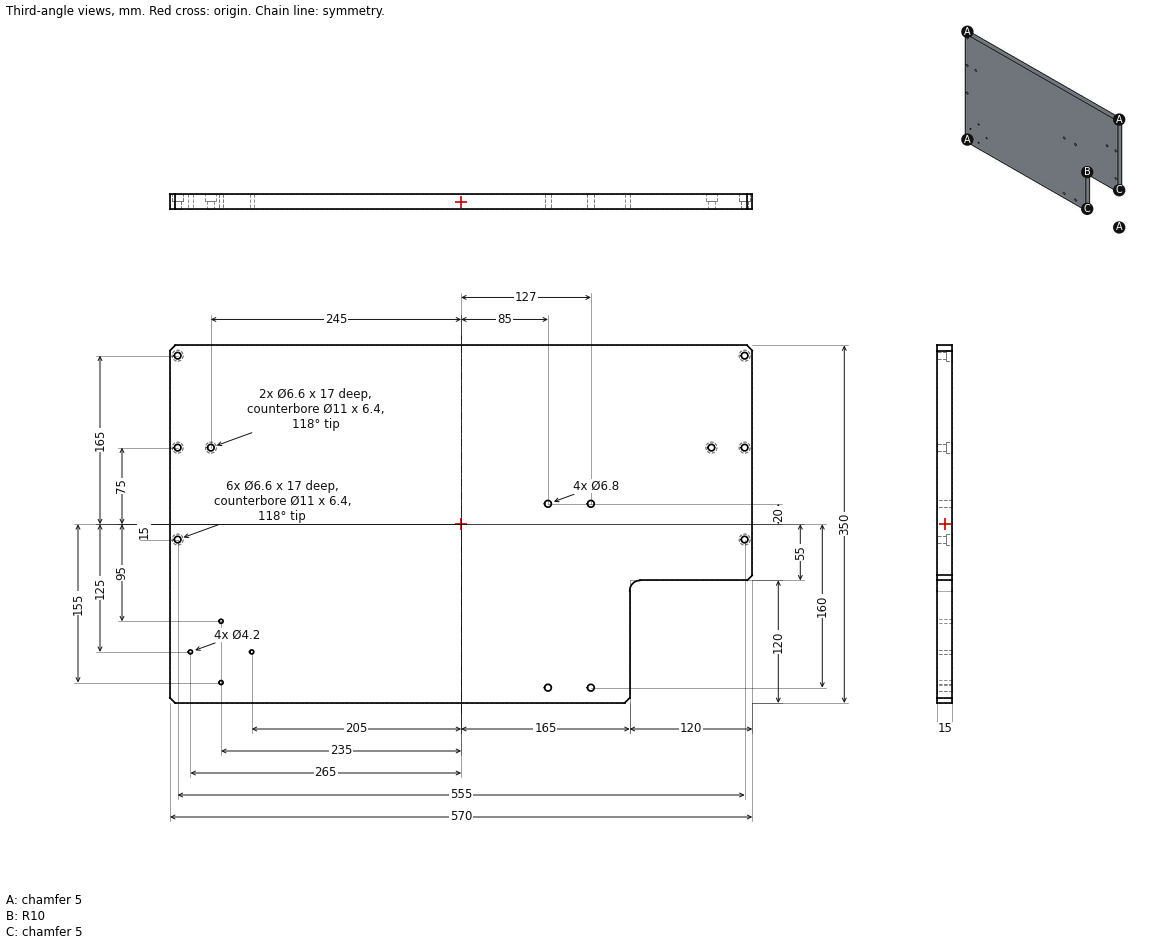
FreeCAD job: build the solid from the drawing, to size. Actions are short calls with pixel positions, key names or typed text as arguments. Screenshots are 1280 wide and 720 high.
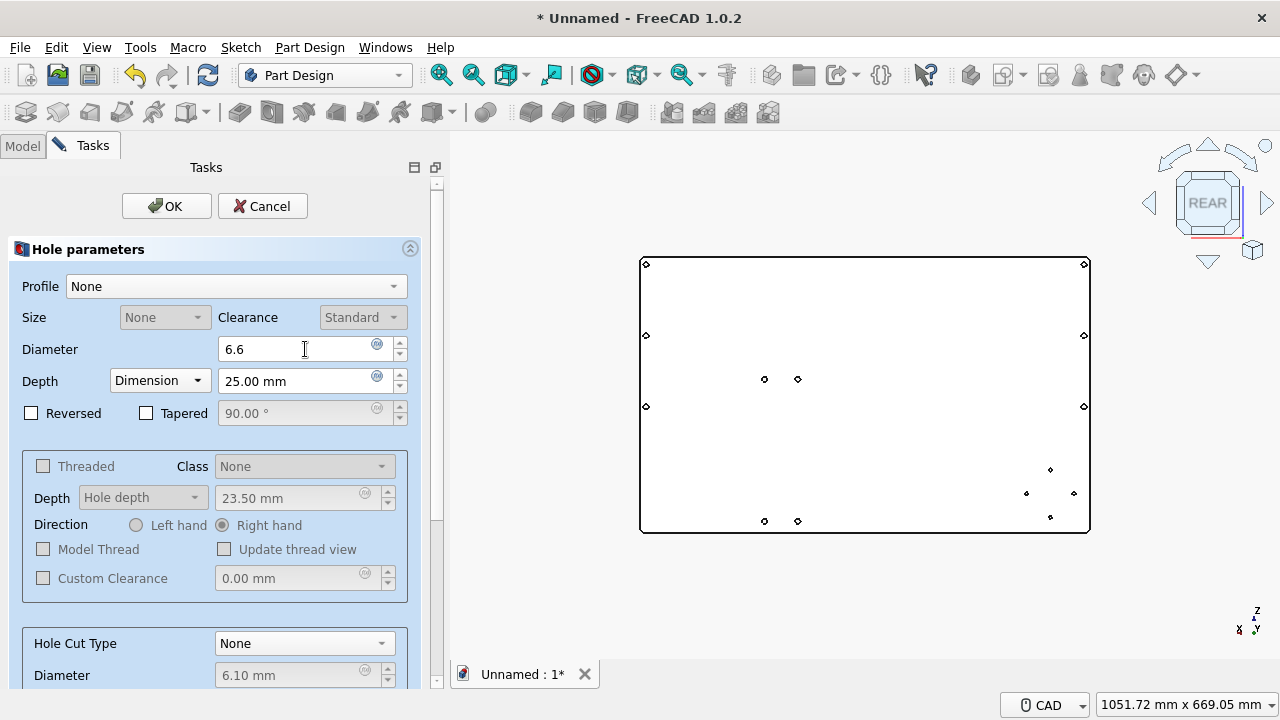
triple_click(305, 381)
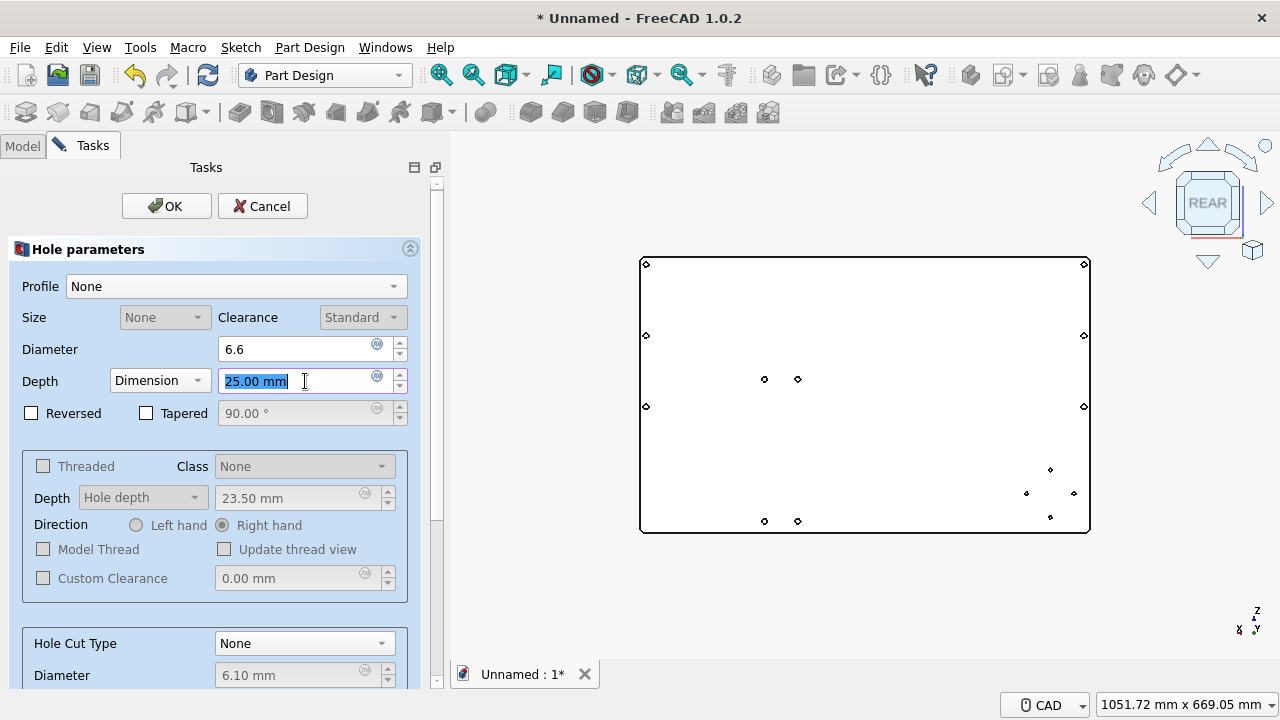
text(17)
key(Tab)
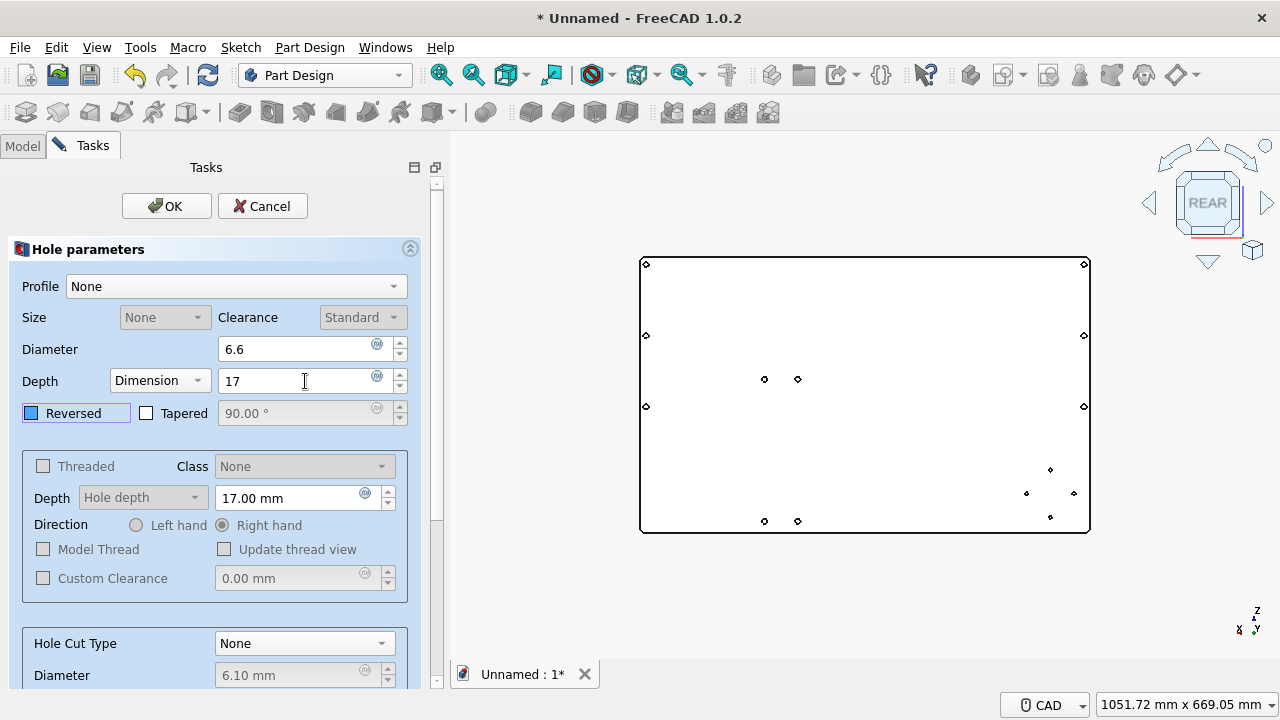
click(306, 644)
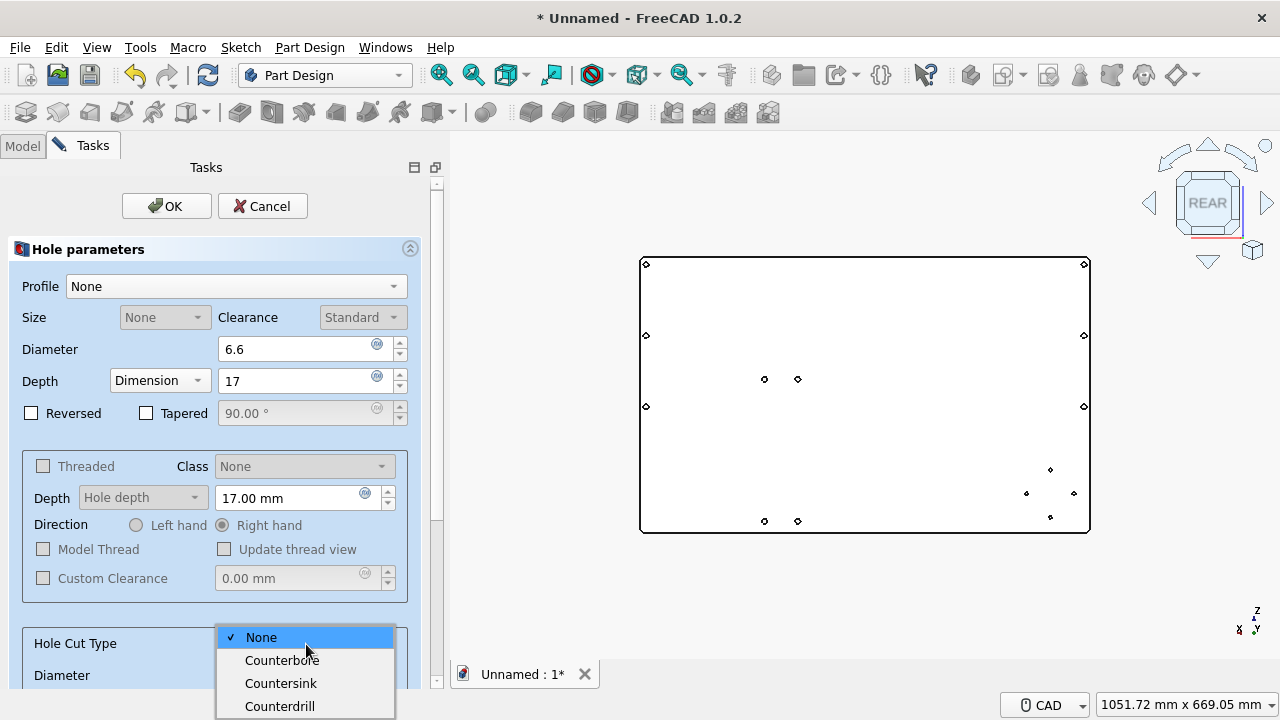
click(304, 660)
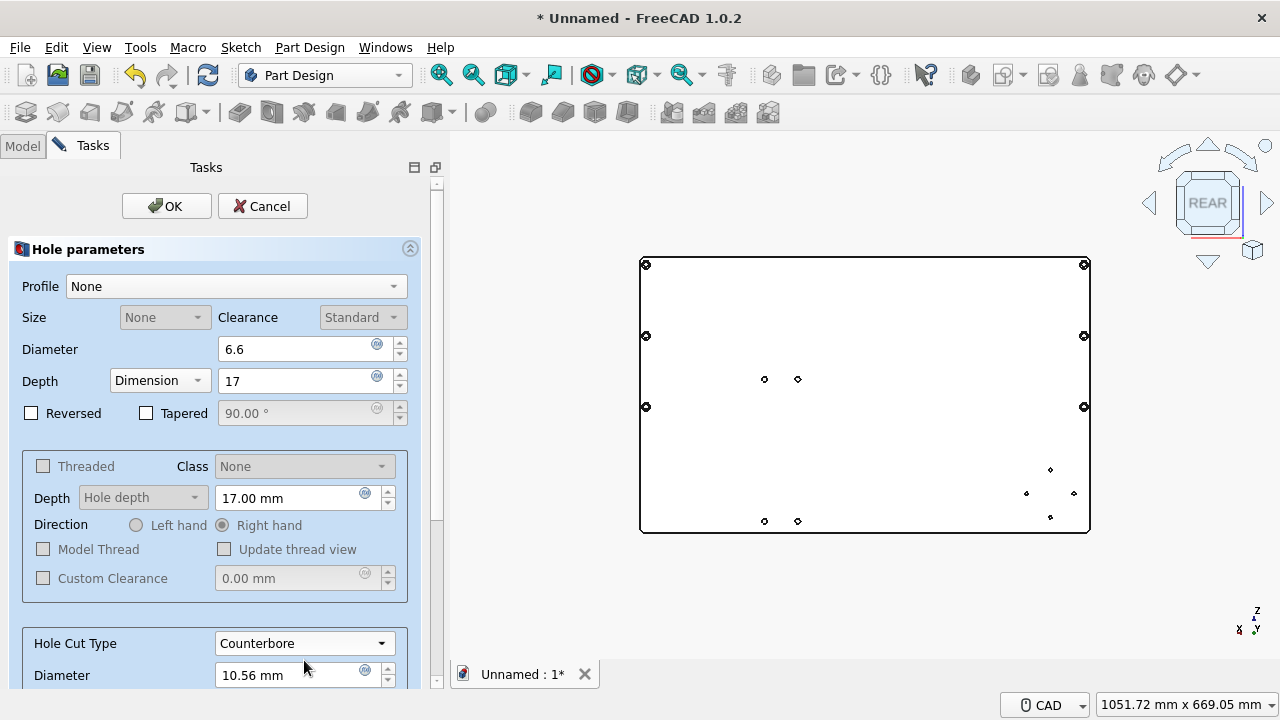
triple_click(298, 675)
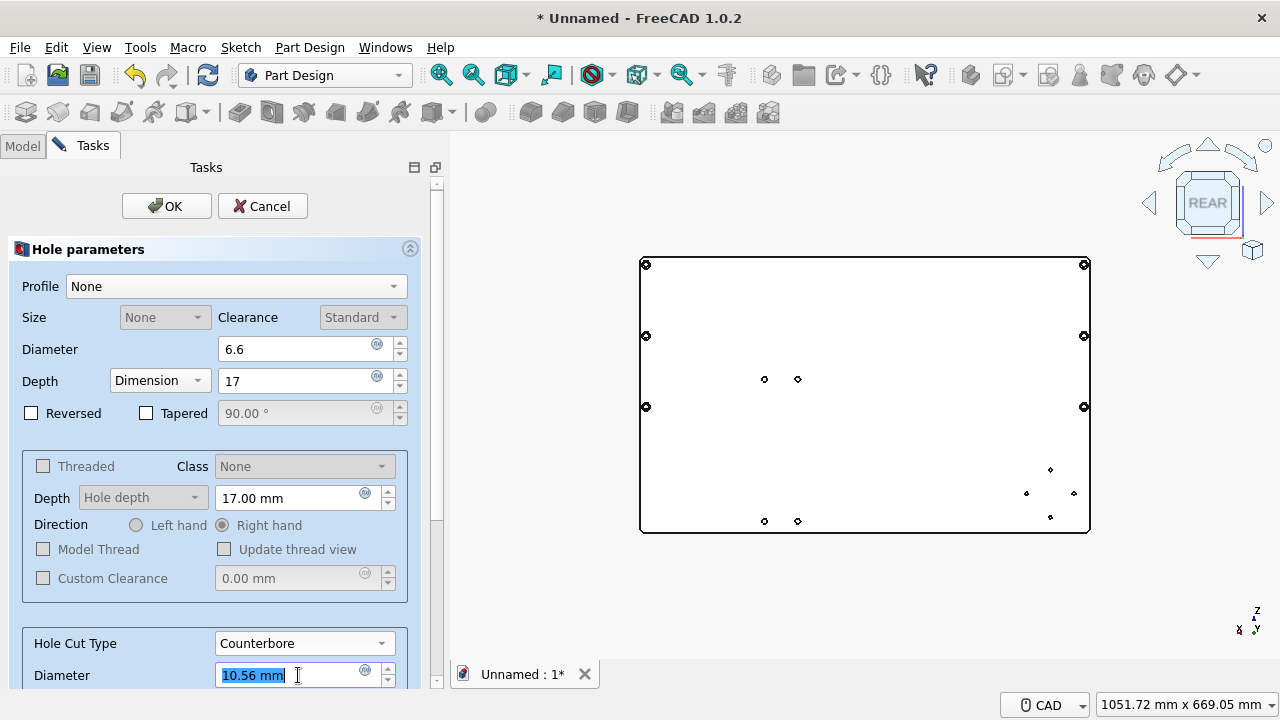
text(11)
key(Tab)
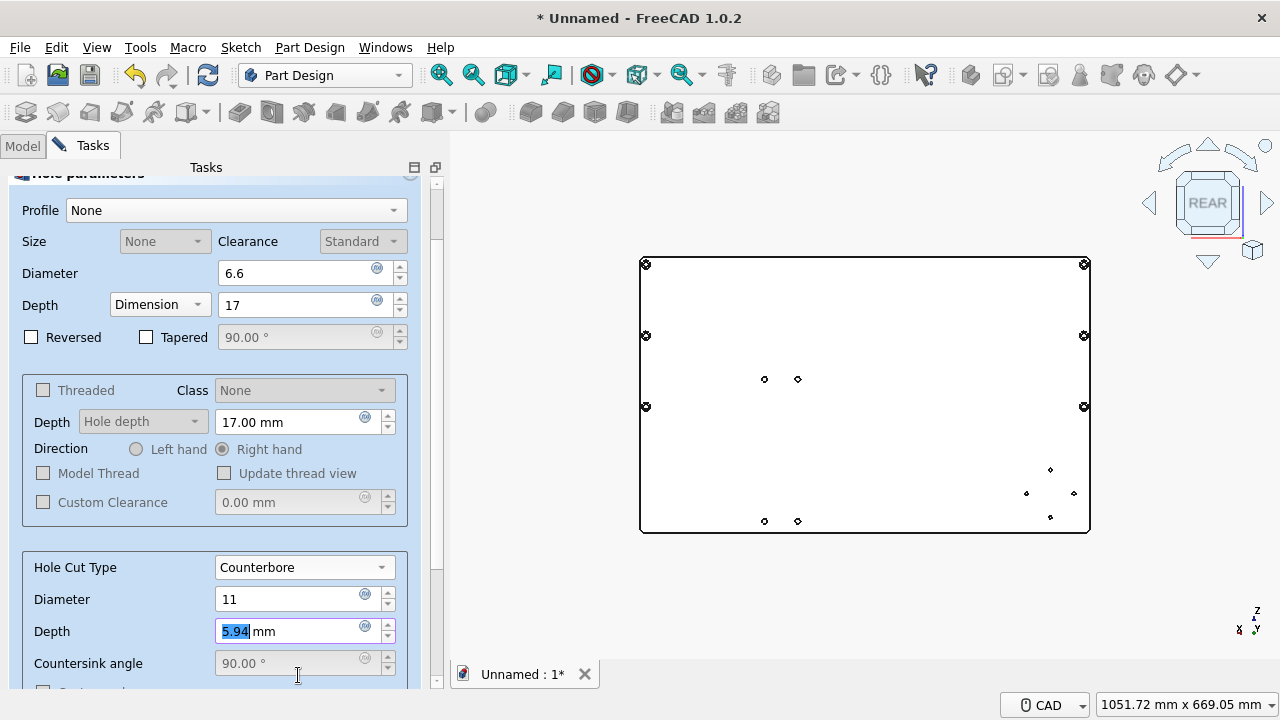
text(6.4)
key(Tab)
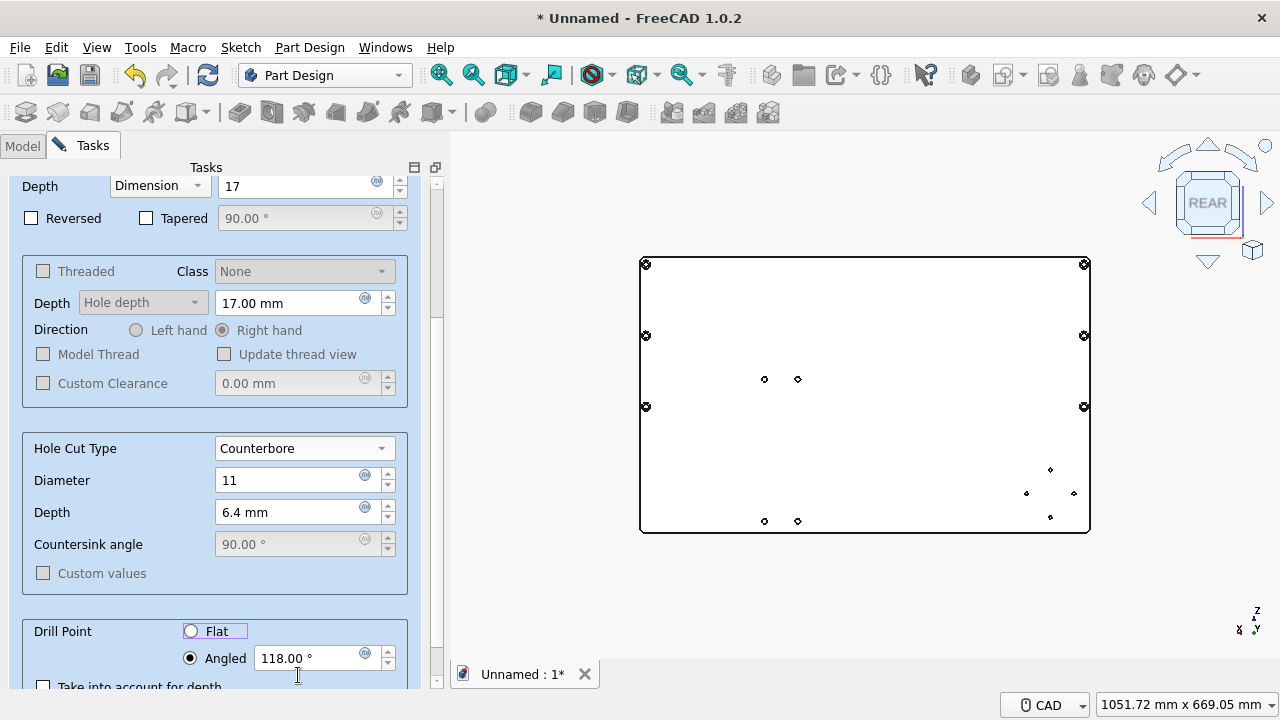
scroll(437, 432, up, 4)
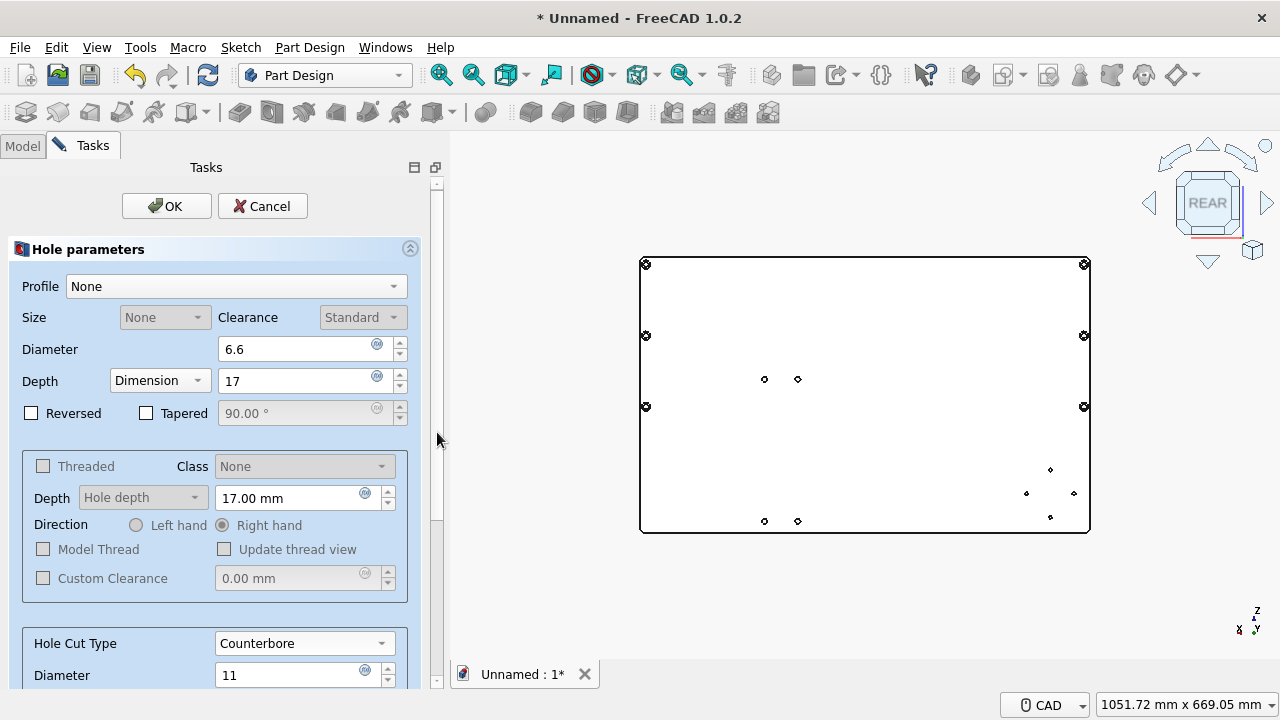
click(167, 206)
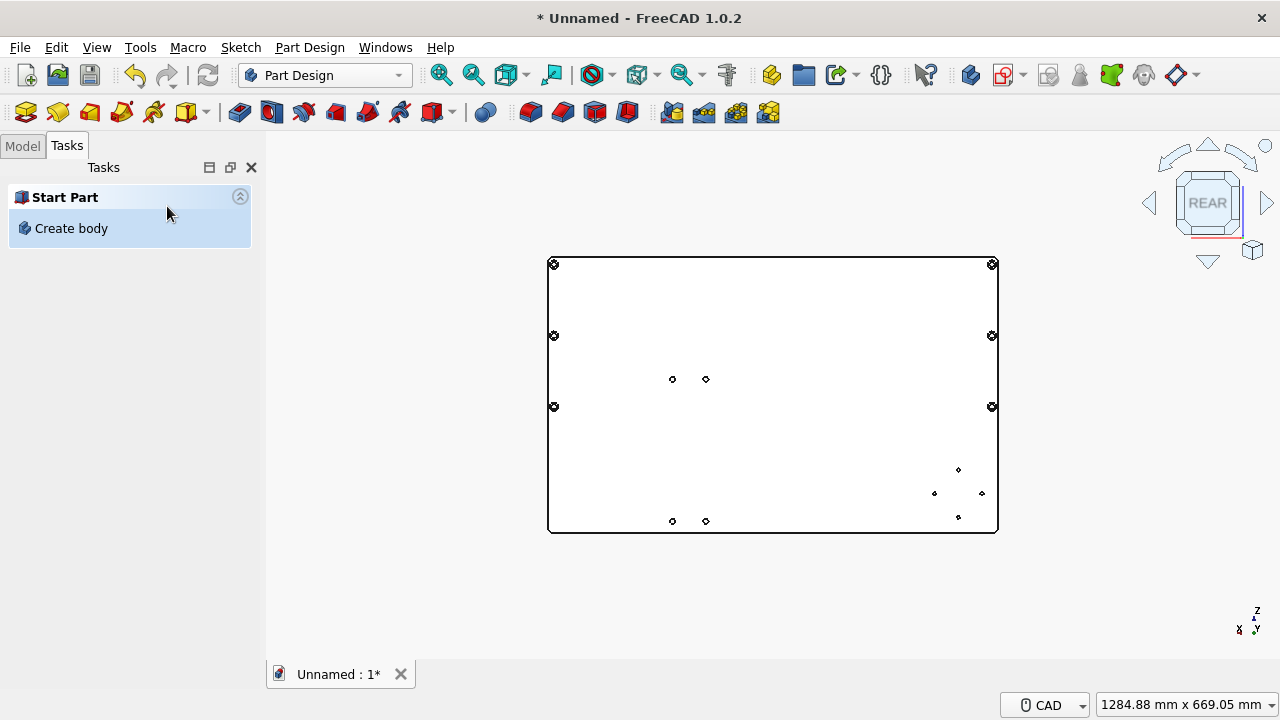
click(837, 394)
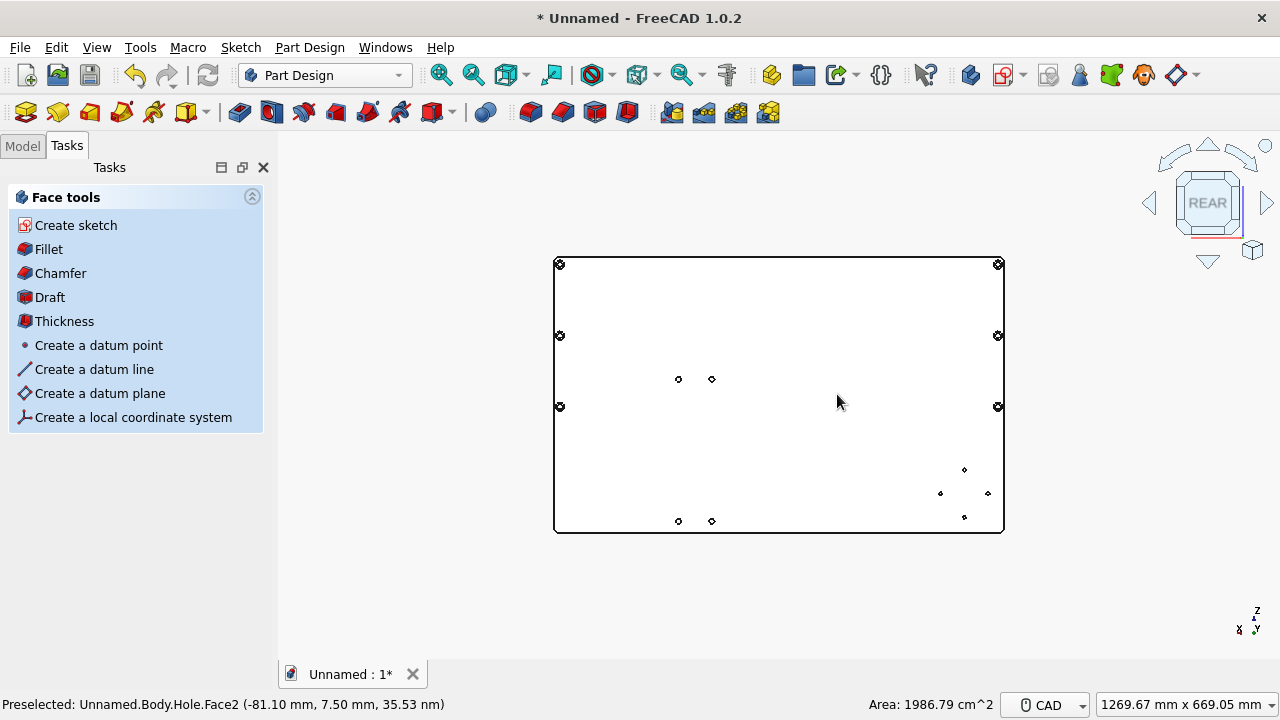
click(1004, 76)